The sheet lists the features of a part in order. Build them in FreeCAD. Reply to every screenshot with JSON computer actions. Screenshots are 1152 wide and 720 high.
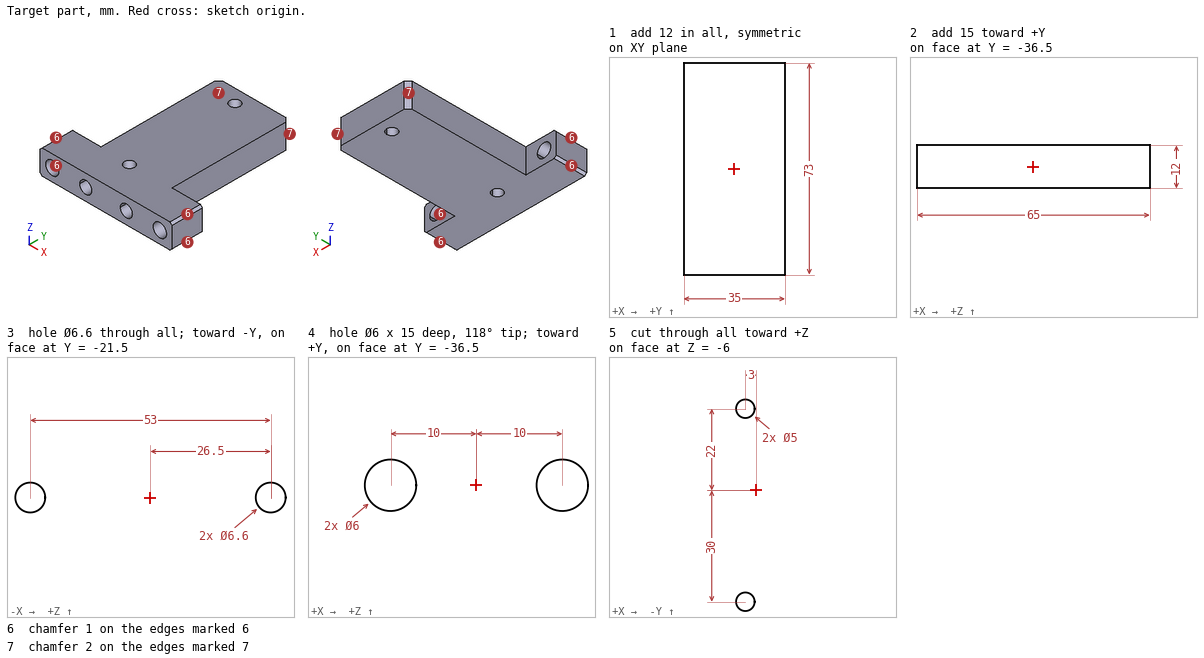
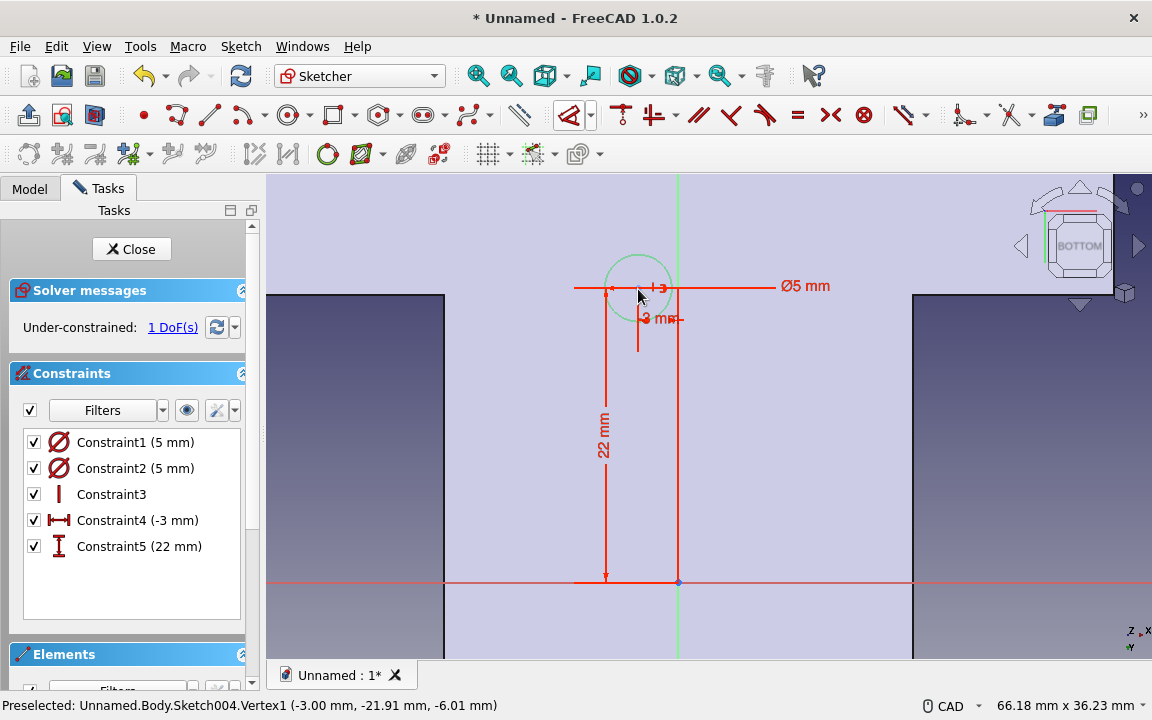
{"action": "scroll", "coordinate": [640, 289], "scroll_direction": "down", "scroll_amount": 5}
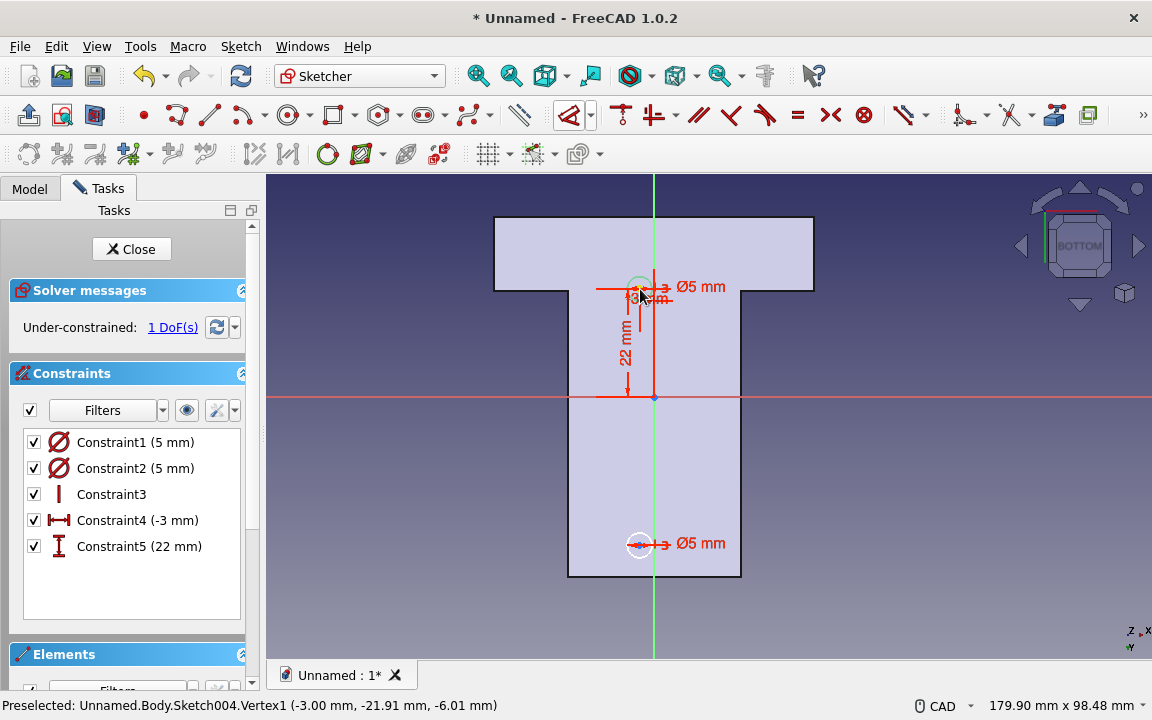
{"action": "left_click", "coordinate": [640, 545]}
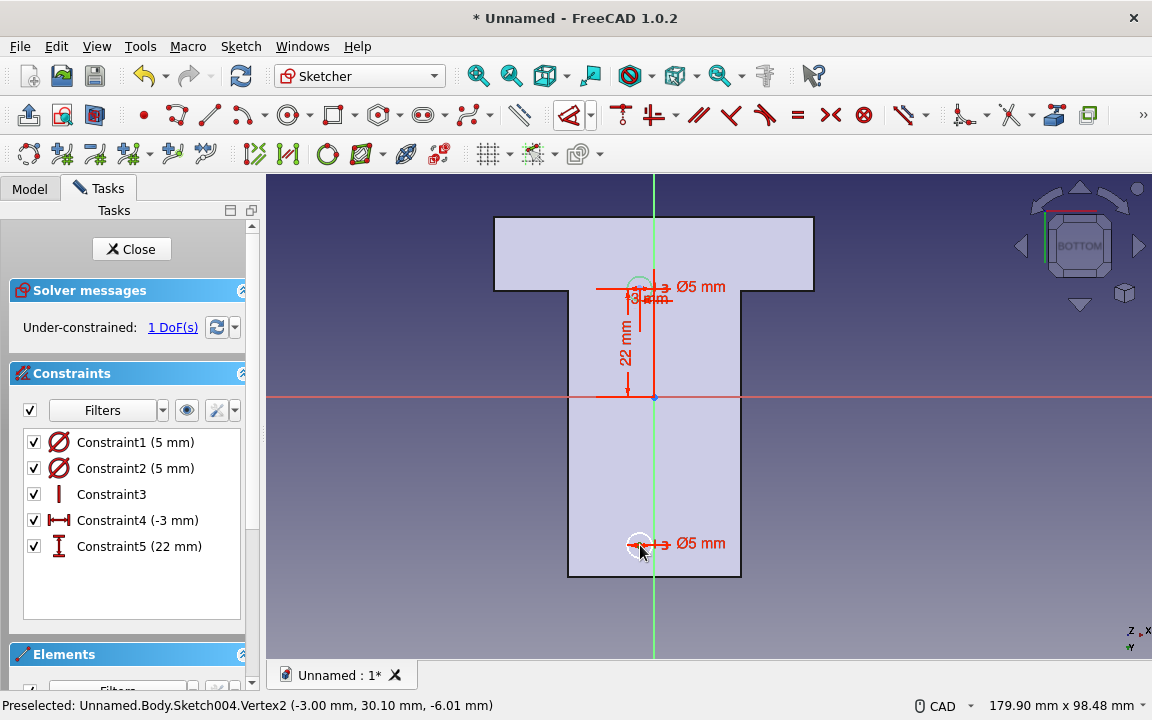
{"action": "key", "text": "i"}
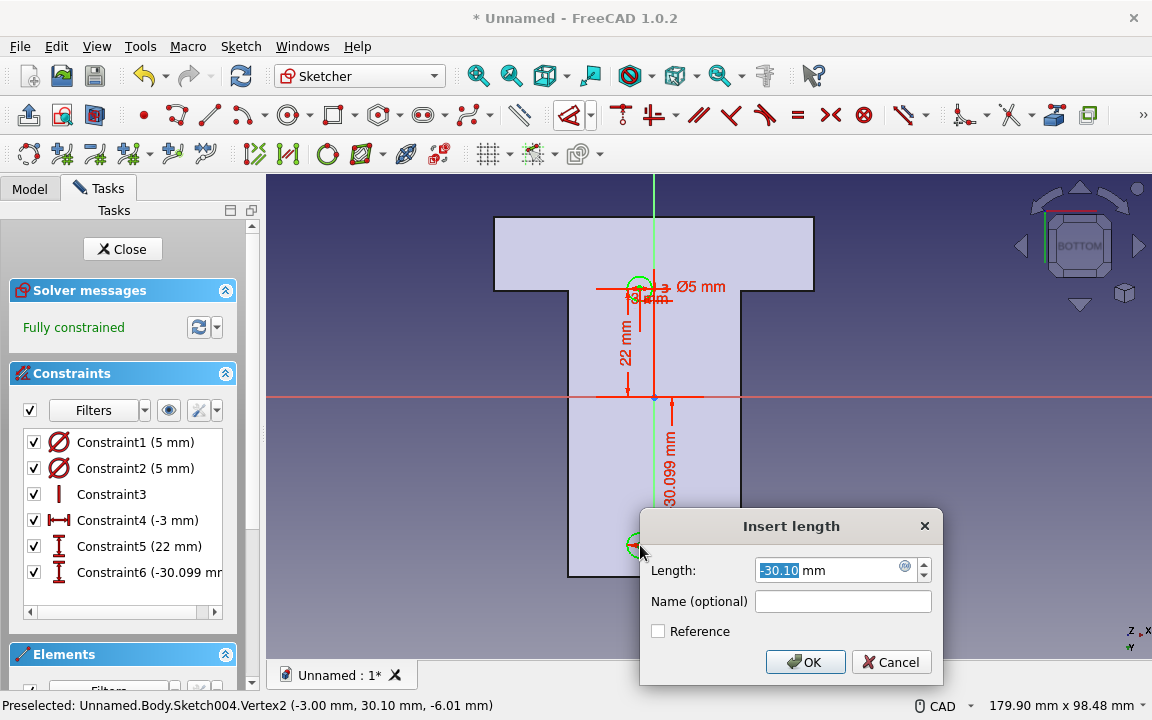
{"action": "type", "text": "-30"}
{"action": "key", "text": "Return"}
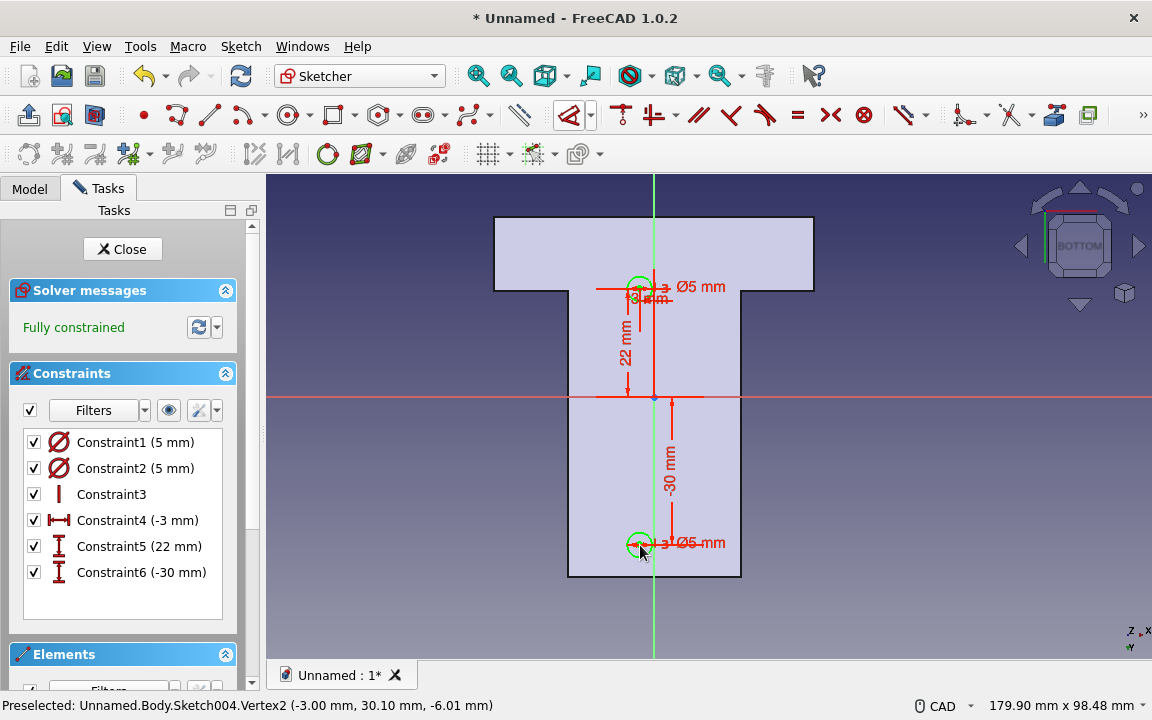
{"action": "left_click", "coordinate": [123, 249]}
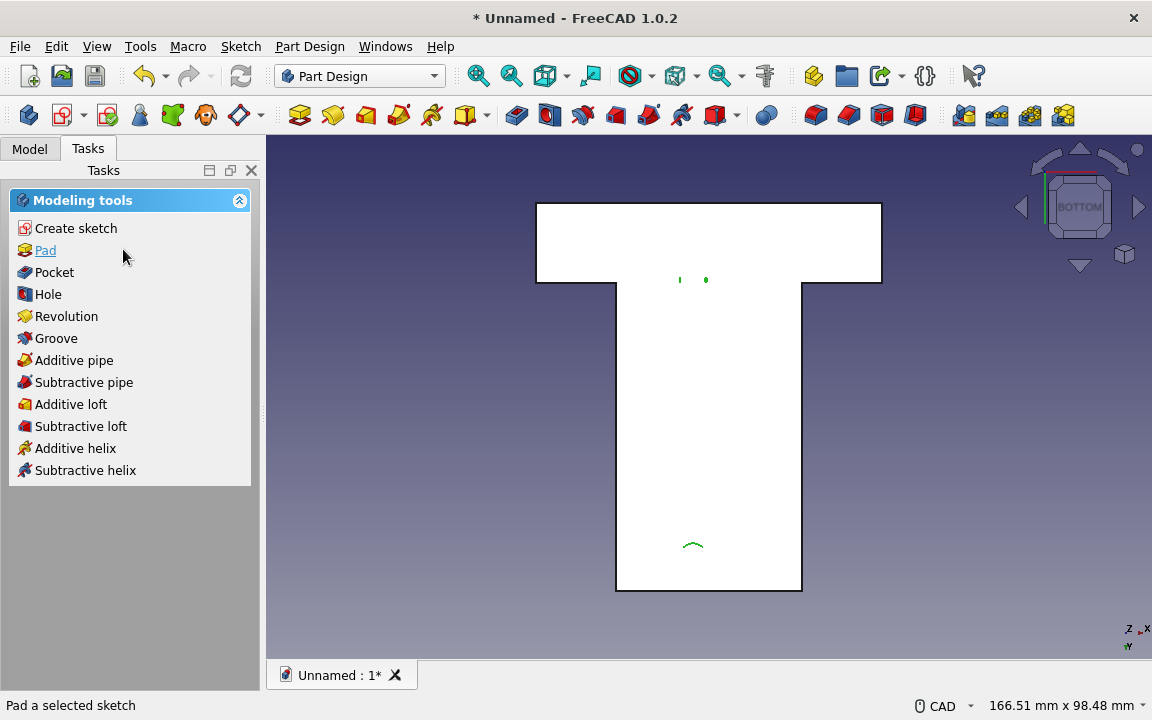
{"action": "left_click", "coordinate": [517, 116]}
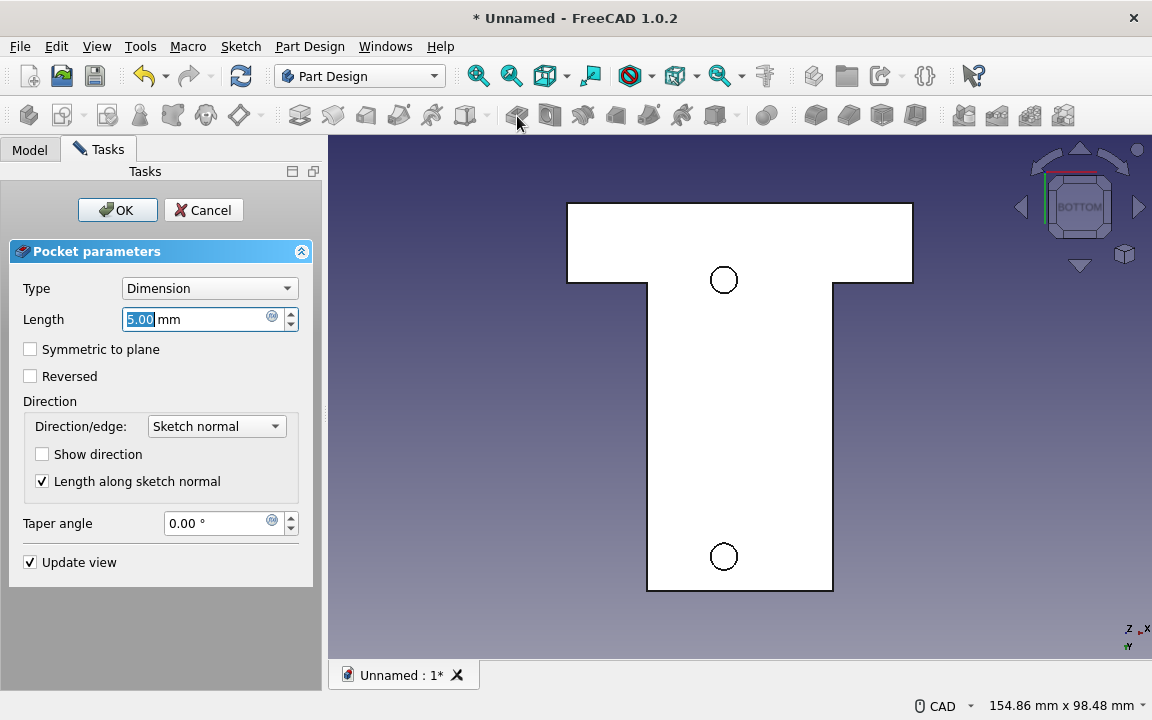
{"action": "left_click", "coordinate": [210, 288]}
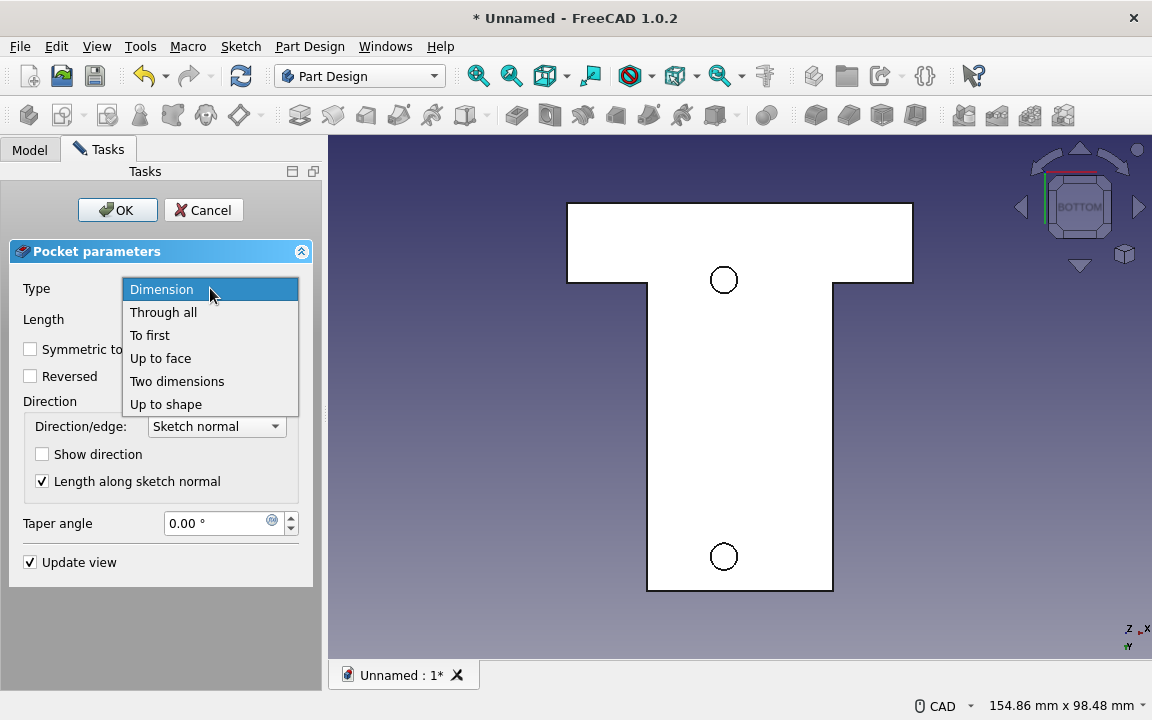
{"action": "left_click", "coordinate": [208, 312]}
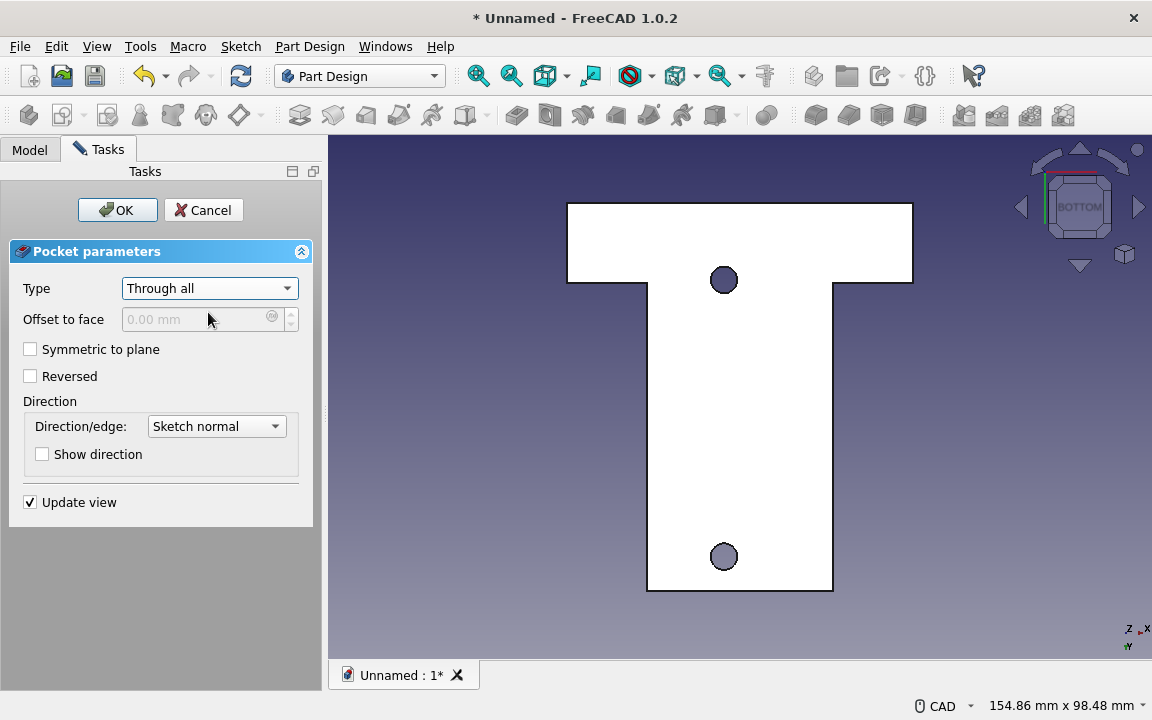
{"action": "left_click", "coordinate": [118, 210]}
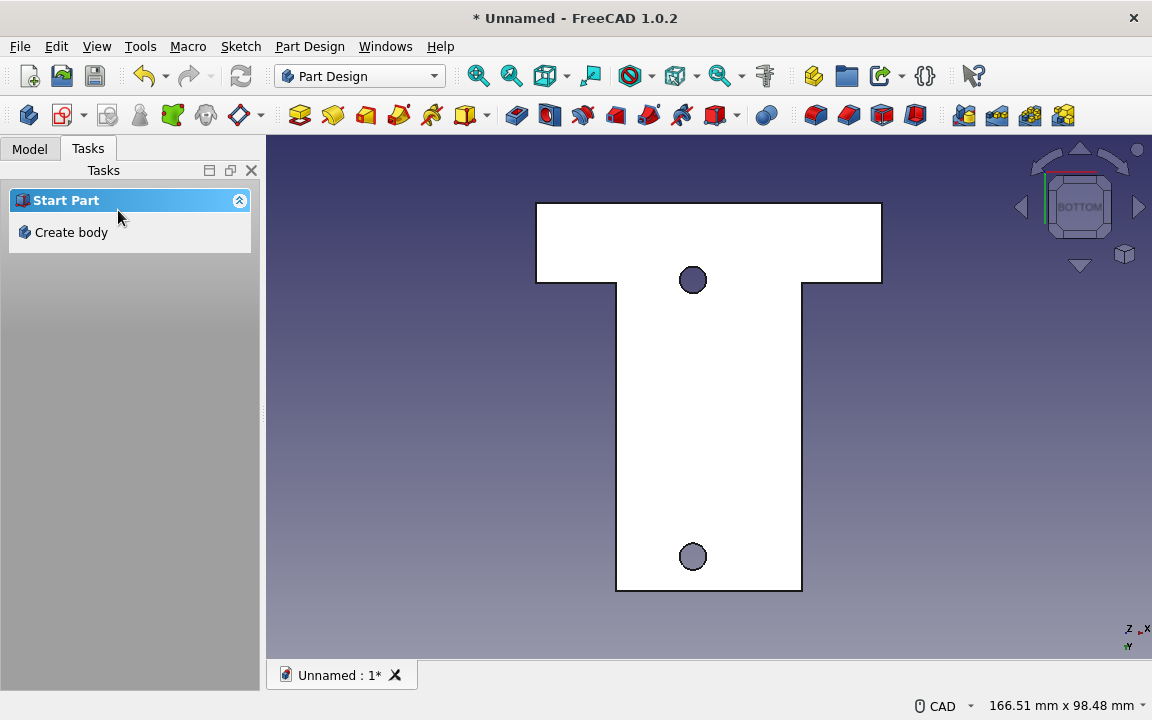
{"action": "left_click", "coordinate": [882, 242]}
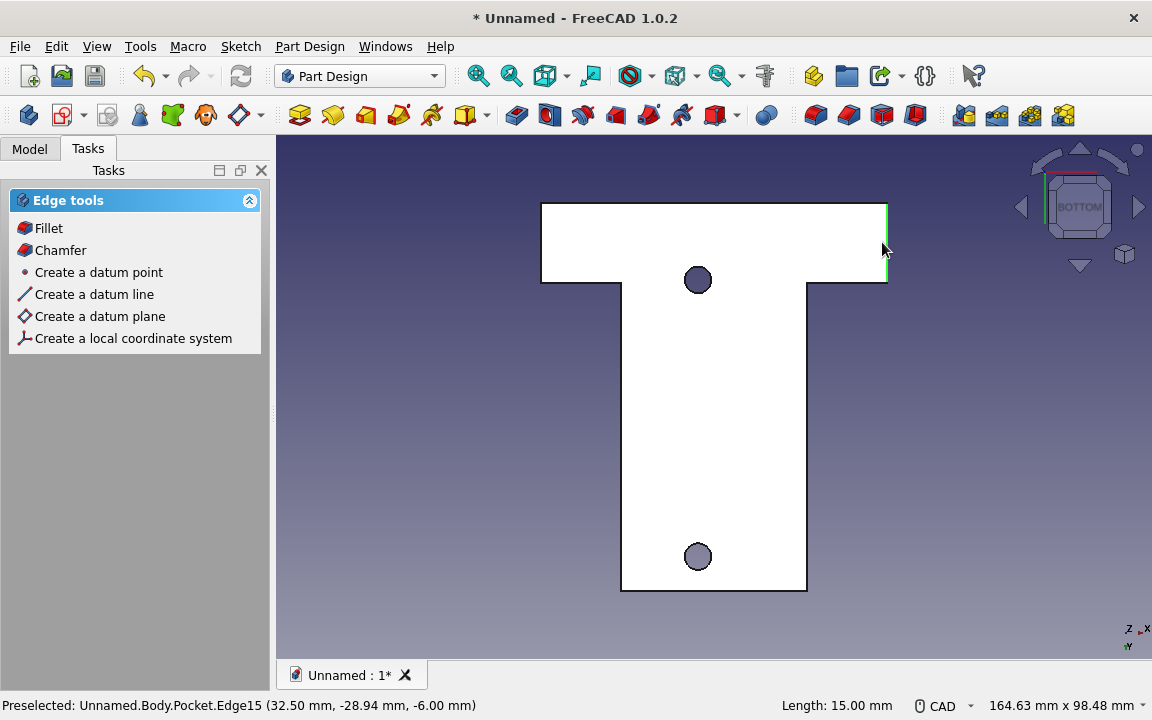
{"action": "left_click", "coordinate": [541, 242], "text": "ctrl"}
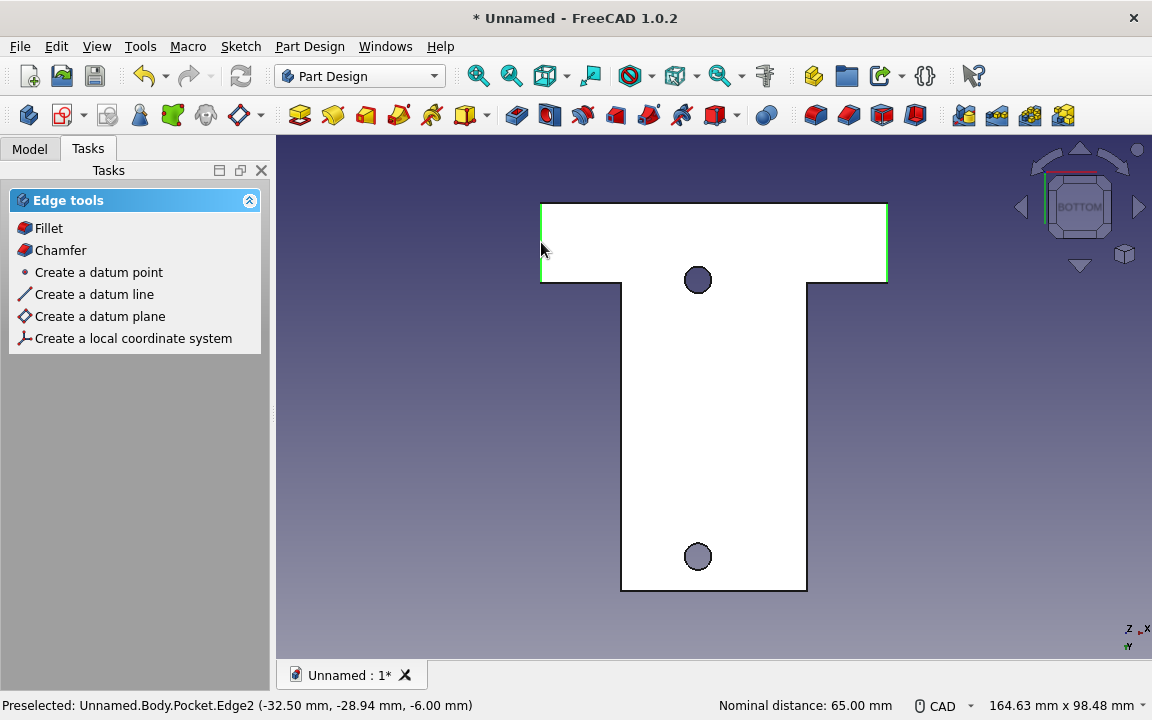
{"action": "key", "text": "0"}